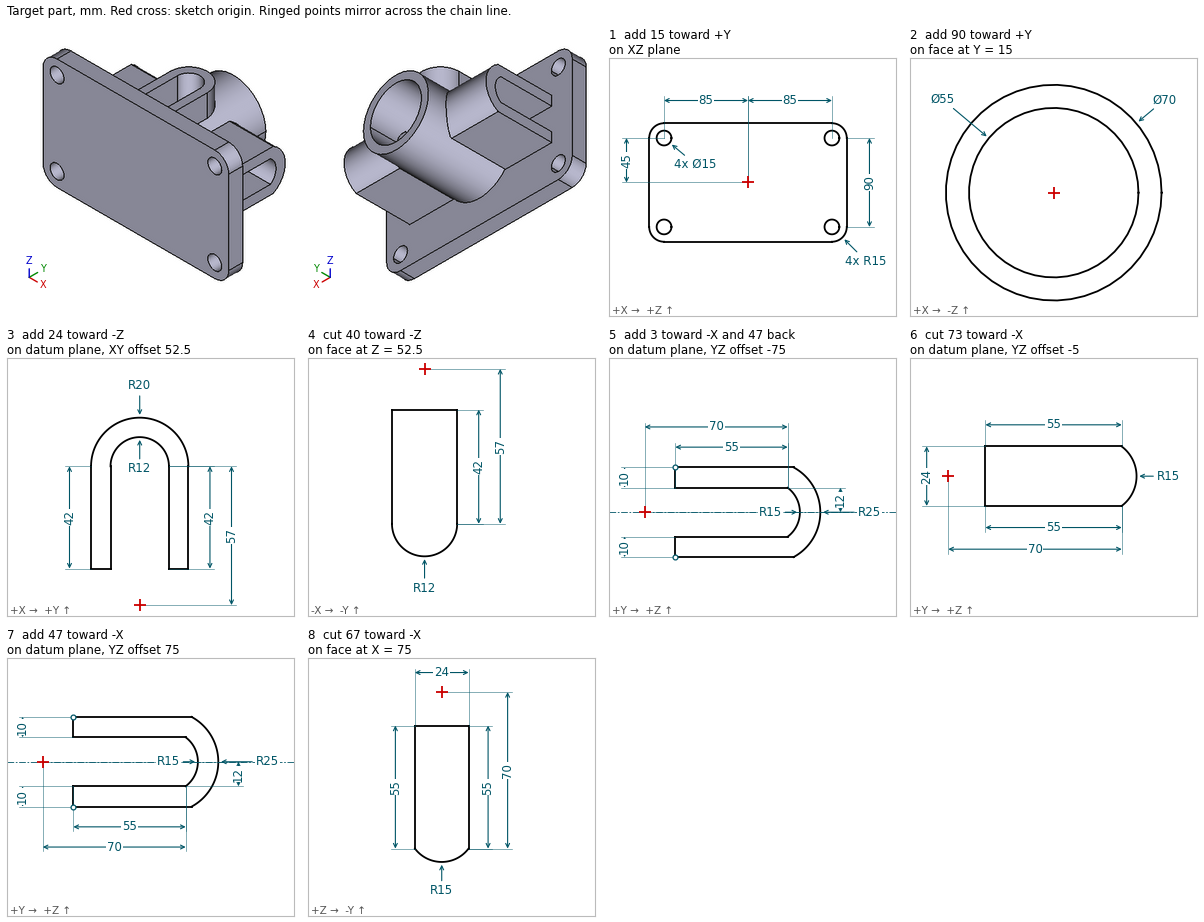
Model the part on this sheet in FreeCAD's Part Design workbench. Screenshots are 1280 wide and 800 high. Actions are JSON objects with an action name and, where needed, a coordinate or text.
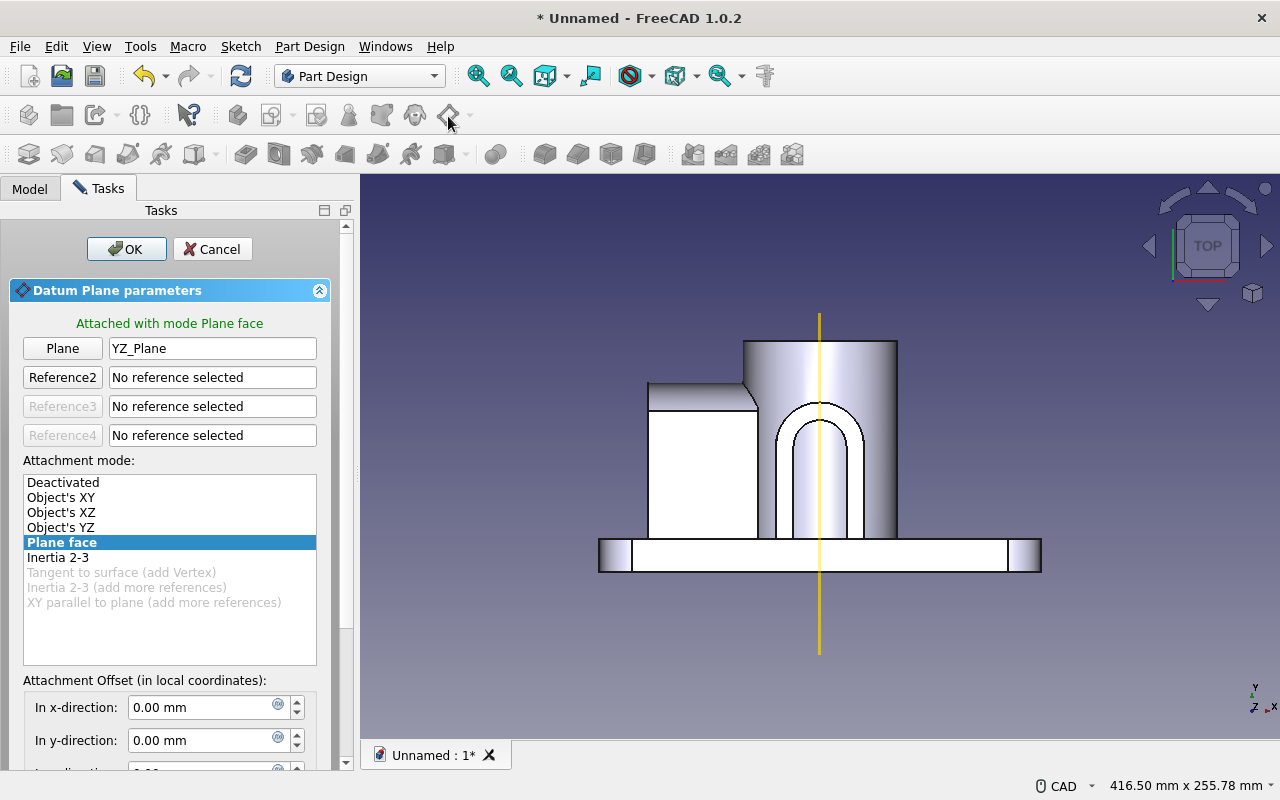
{"action": "scroll", "coordinate": [346, 495], "scroll_direction": "down", "scroll_amount": 2}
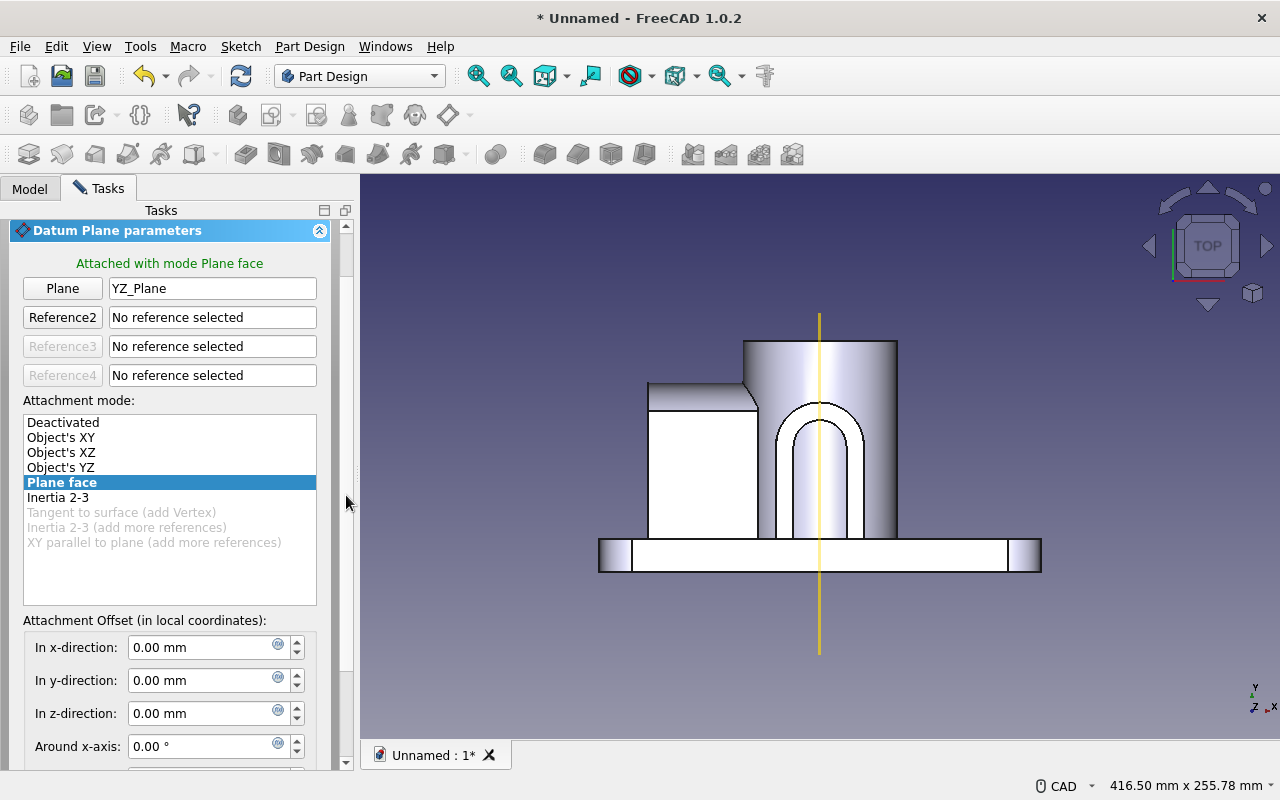
{"action": "triple_click", "coordinate": [210, 654]}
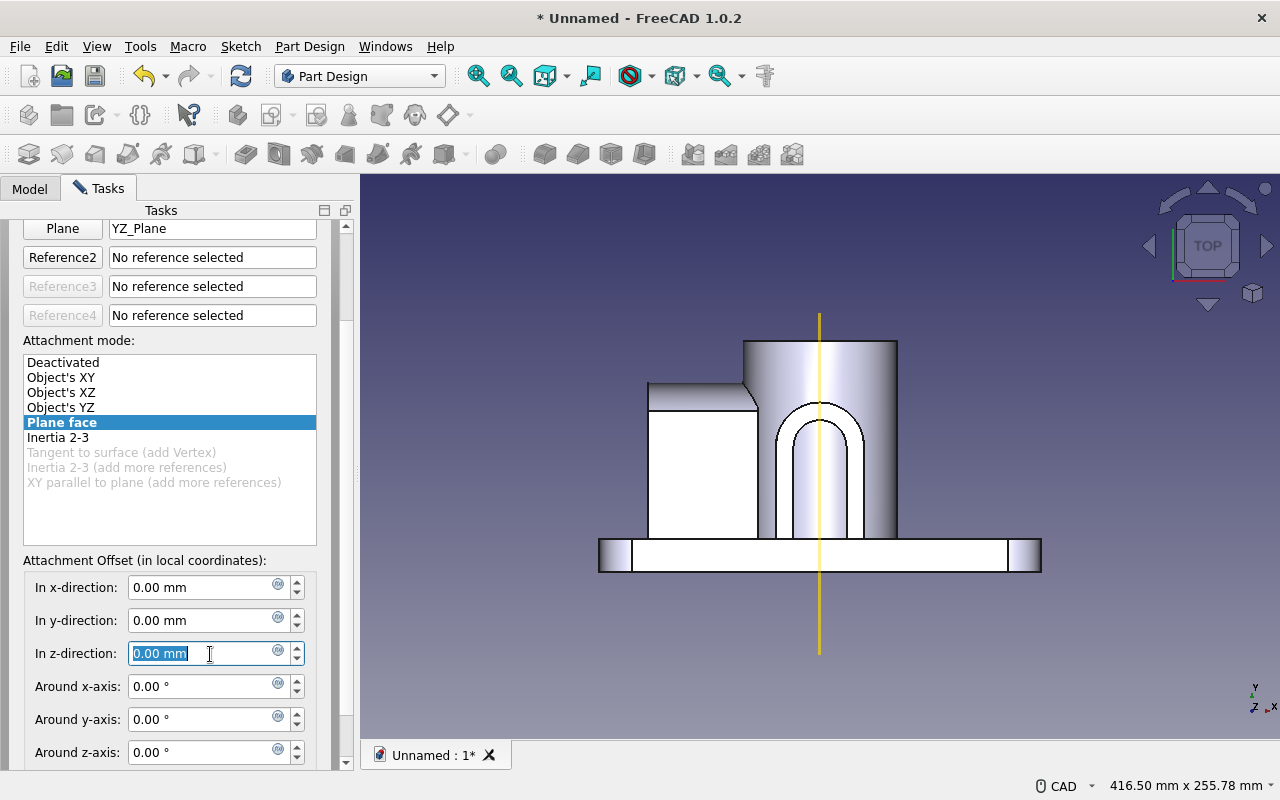
{"action": "type", "text": "-5"}
{"action": "key", "text": "Tab"}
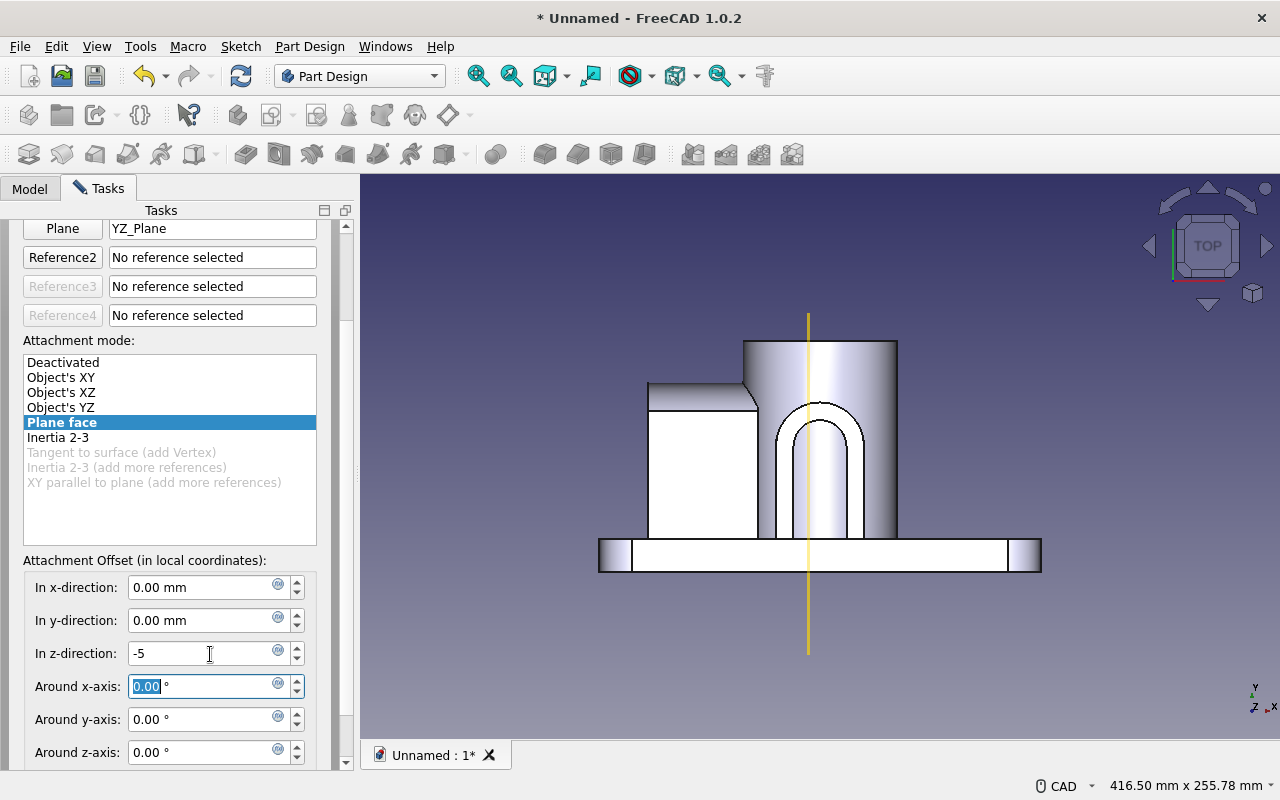
{"action": "scroll", "coordinate": [346, 495], "scroll_direction": "up", "scroll_amount": 3}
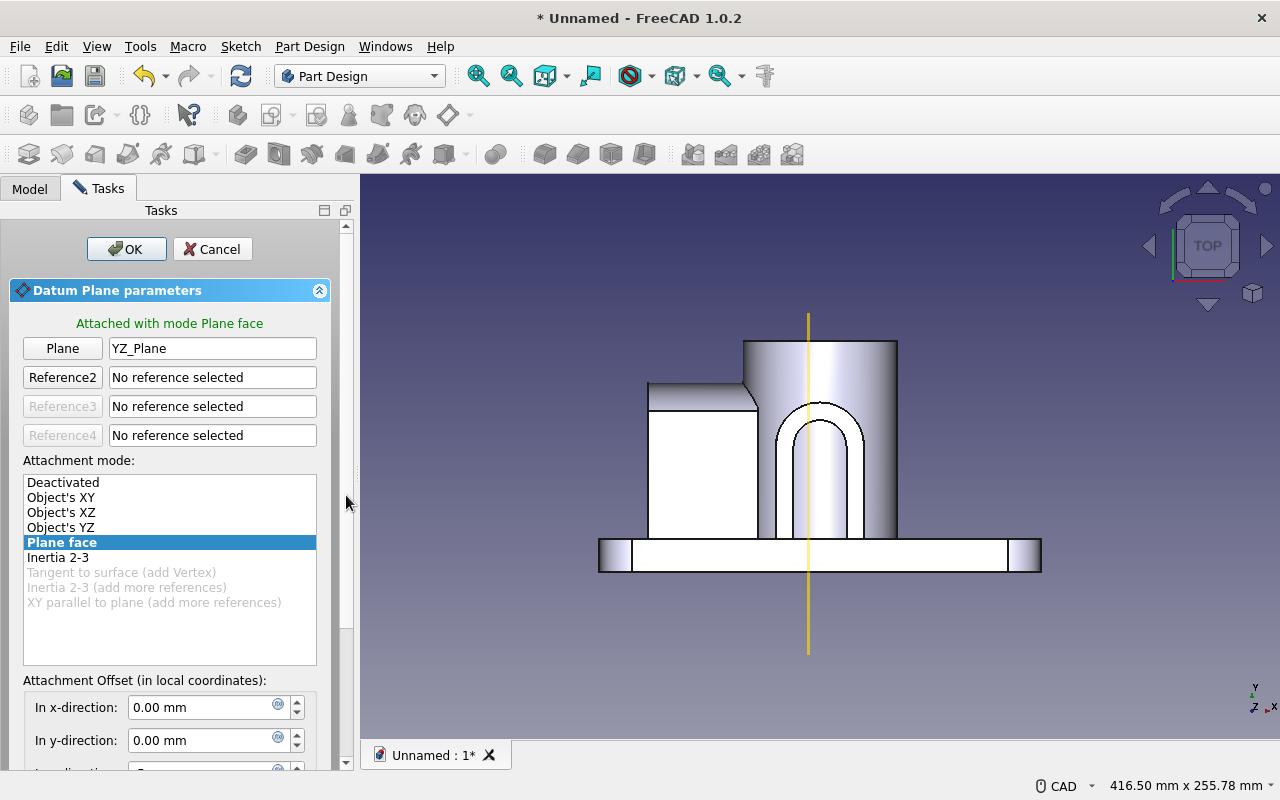
{"action": "left_click", "coordinate": [127, 249]}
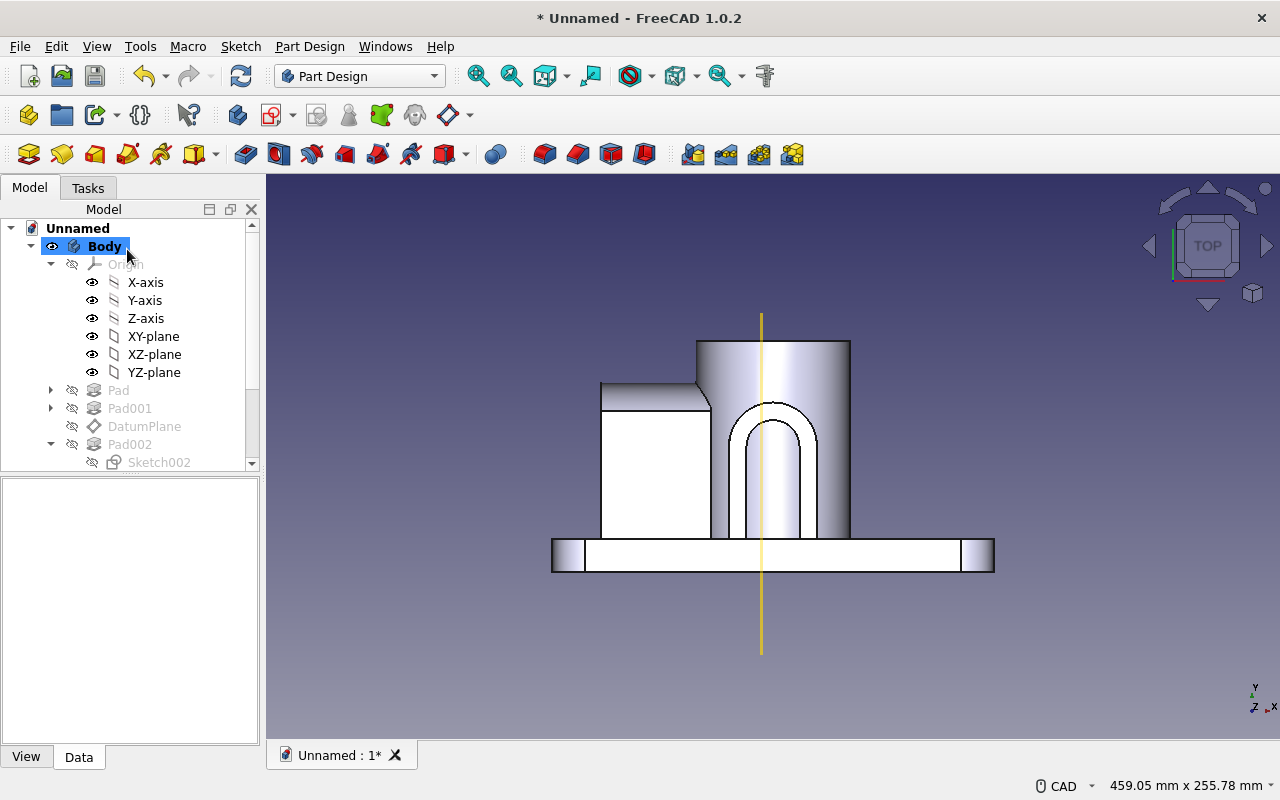
{"action": "scroll", "coordinate": [101, 350], "scroll_direction": "down", "scroll_amount": 3}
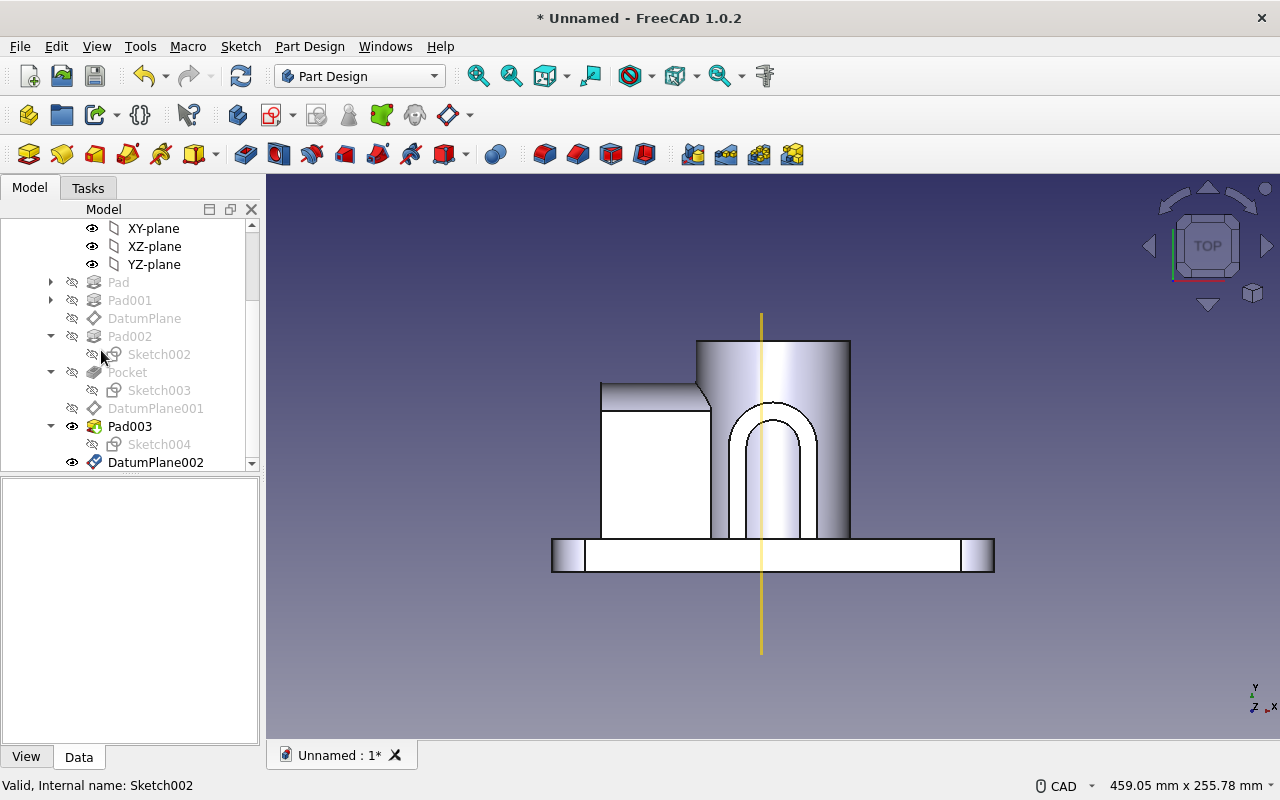
{"action": "left_click", "coordinate": [117, 462]}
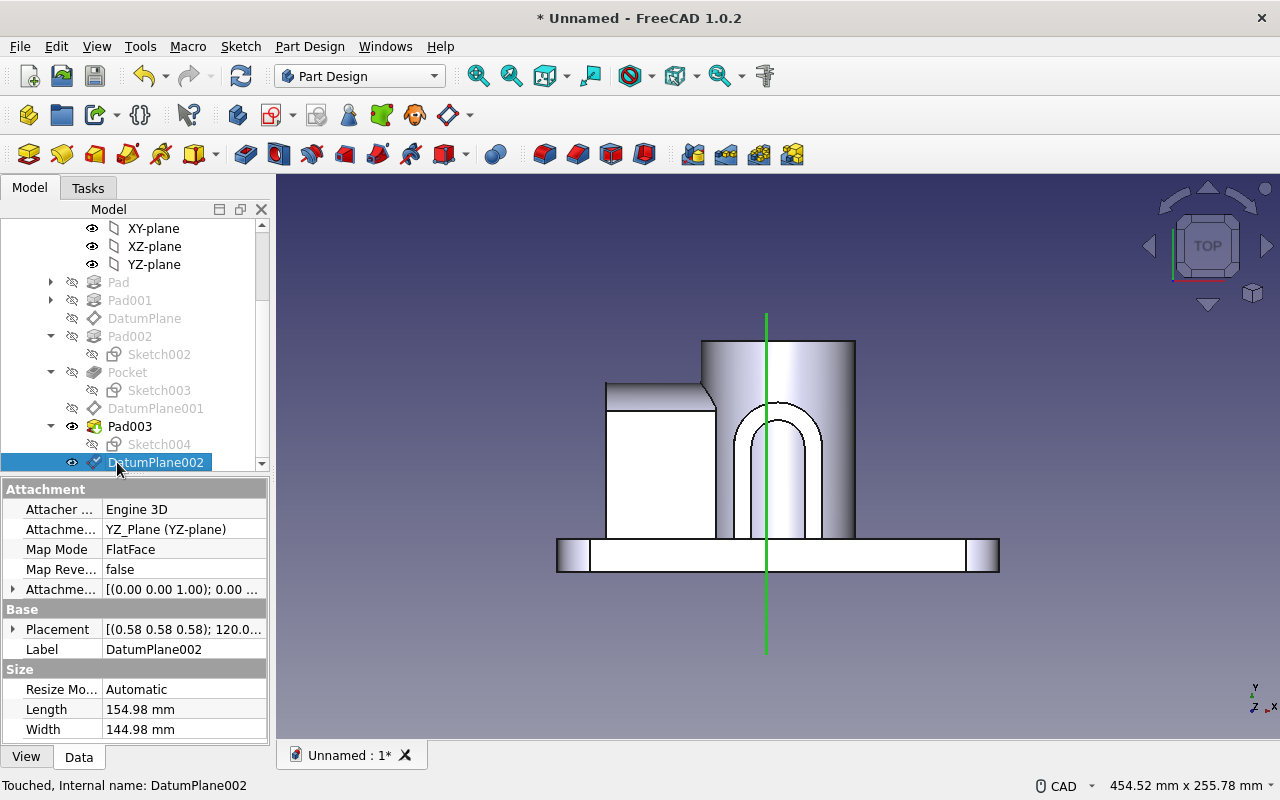
{"action": "left_click", "coordinate": [270, 116]}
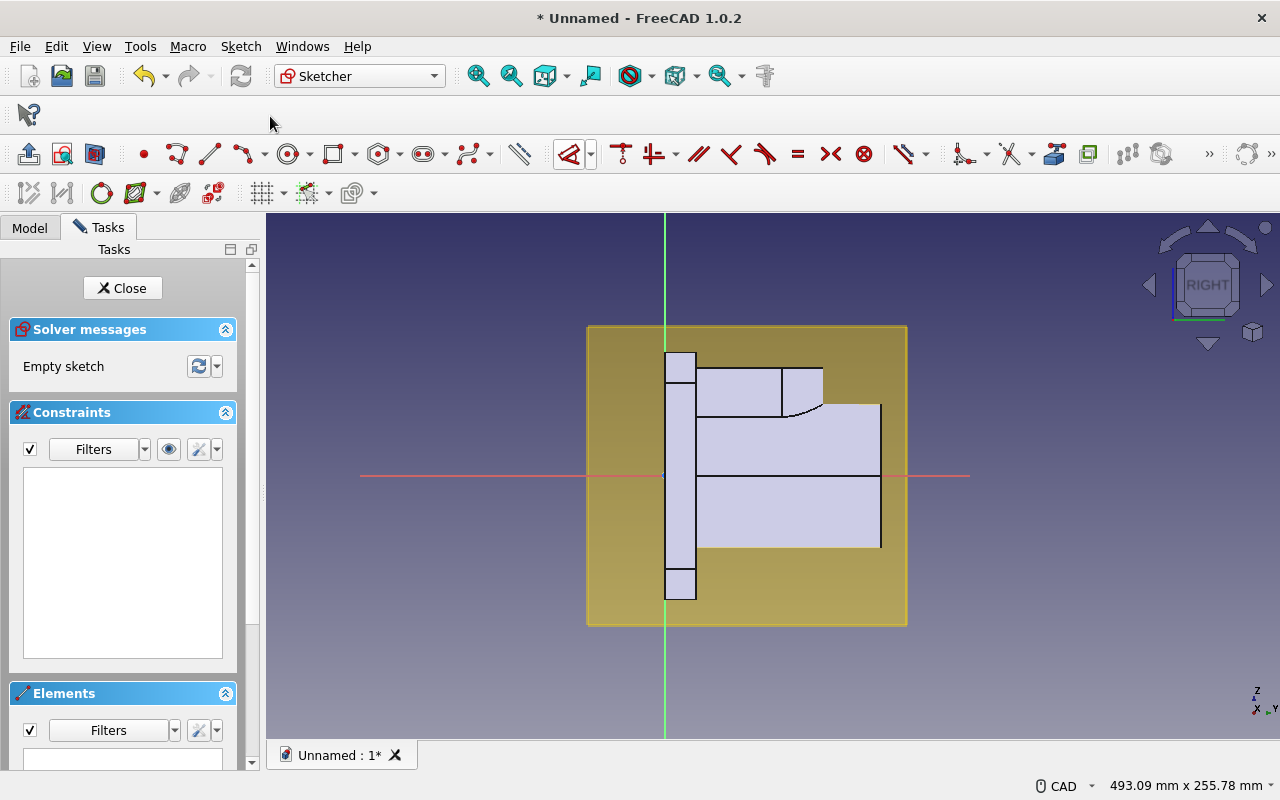
{"action": "key", "text": "q s"}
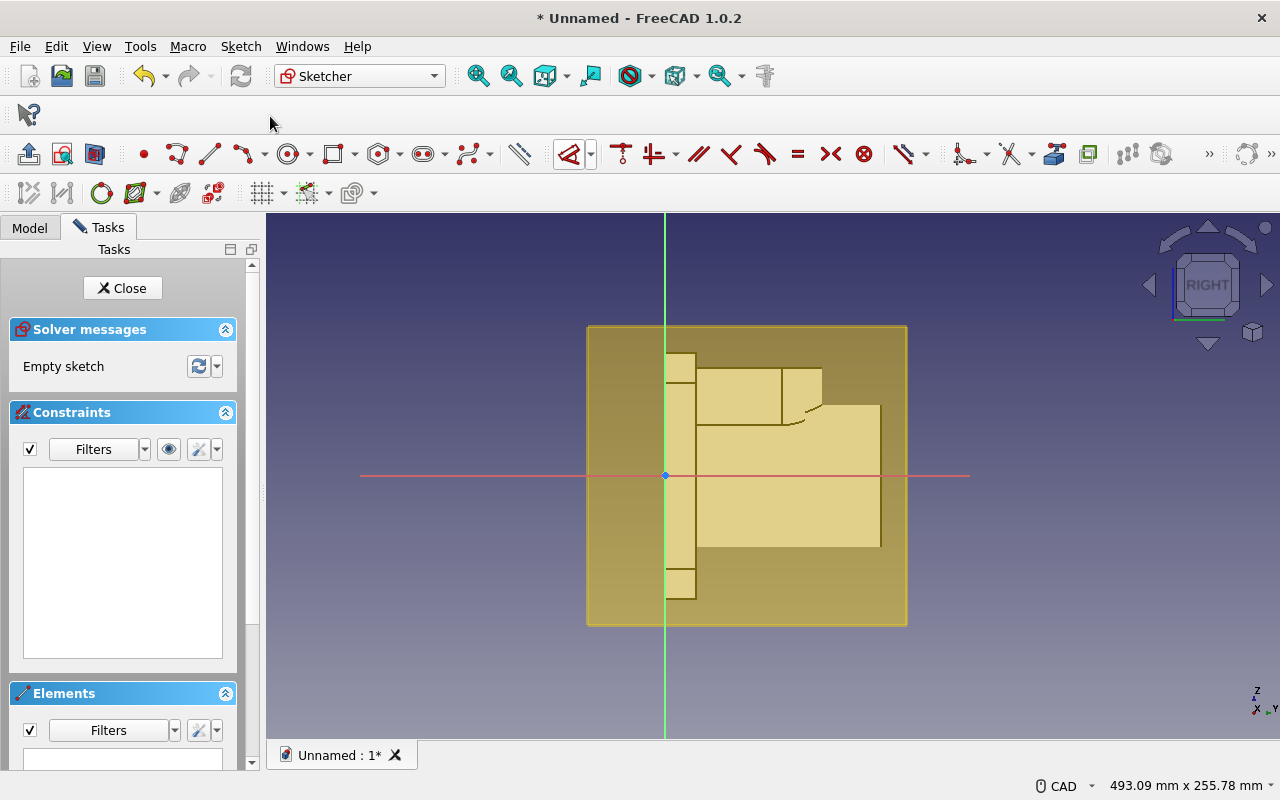
{"action": "scroll", "coordinate": [756, 476], "scroll_direction": "up", "scroll_amount": 7}